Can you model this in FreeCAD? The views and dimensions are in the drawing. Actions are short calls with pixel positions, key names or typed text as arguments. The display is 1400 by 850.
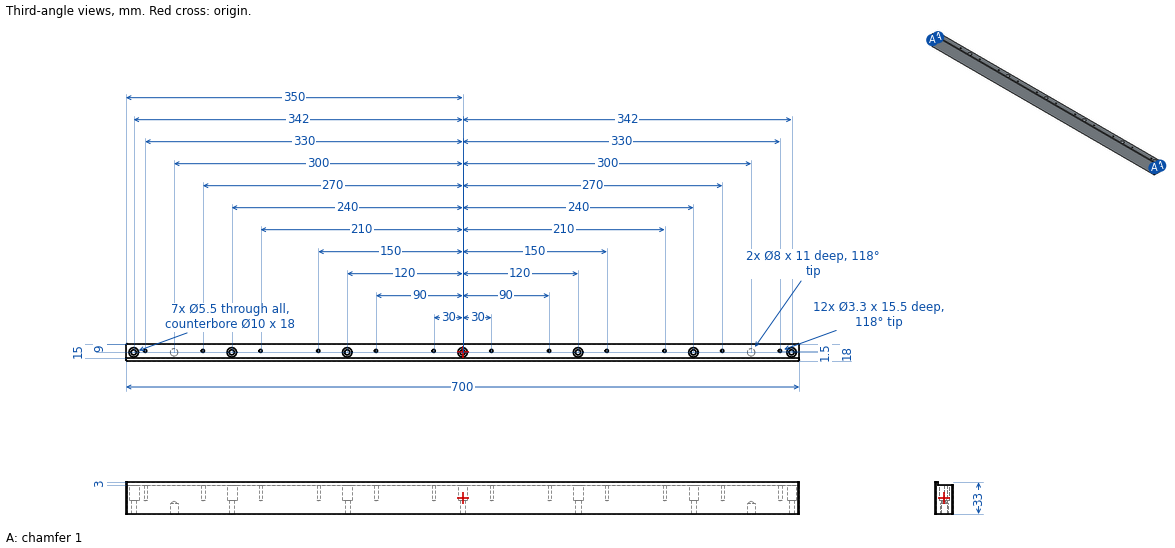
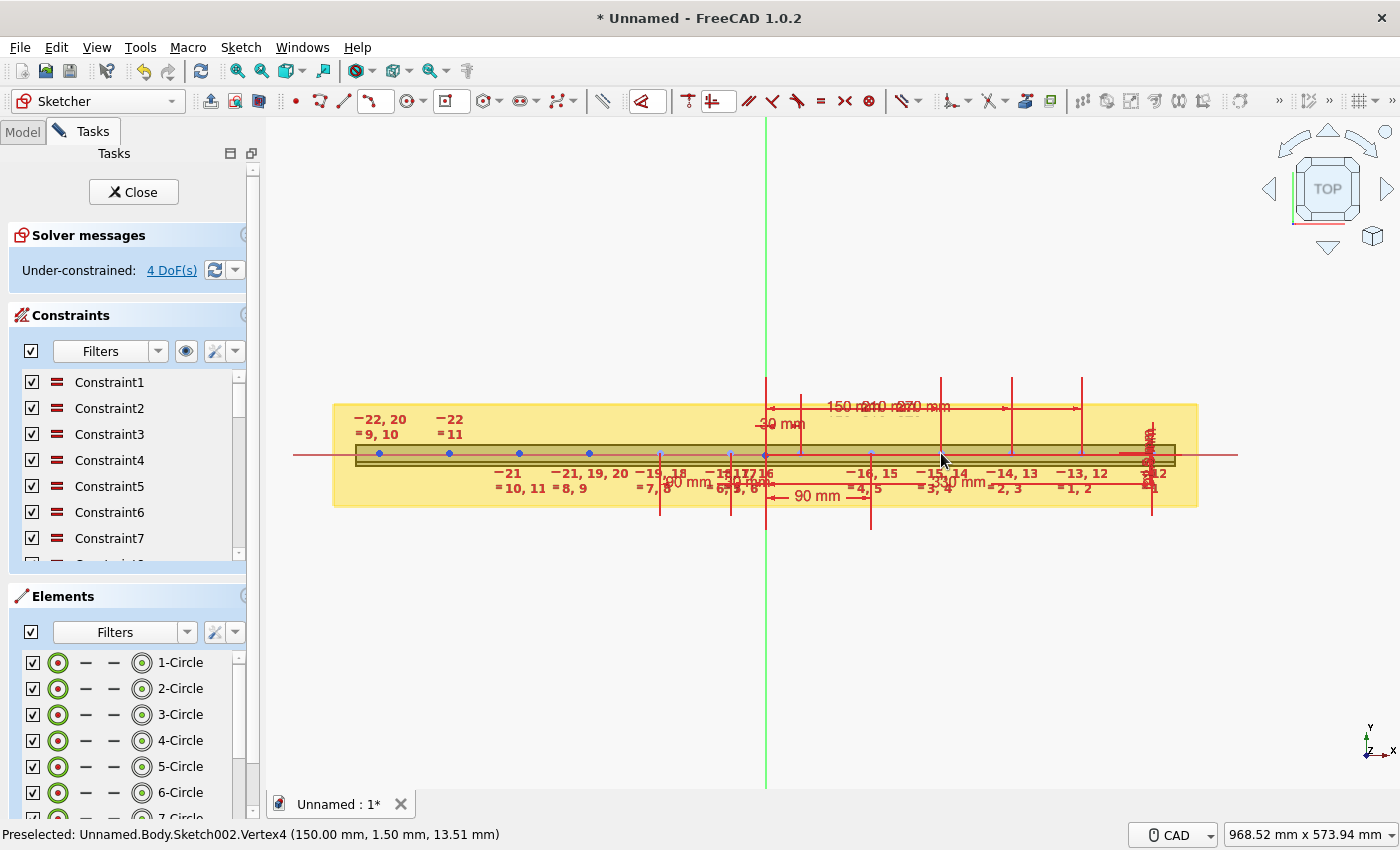
click(590, 453)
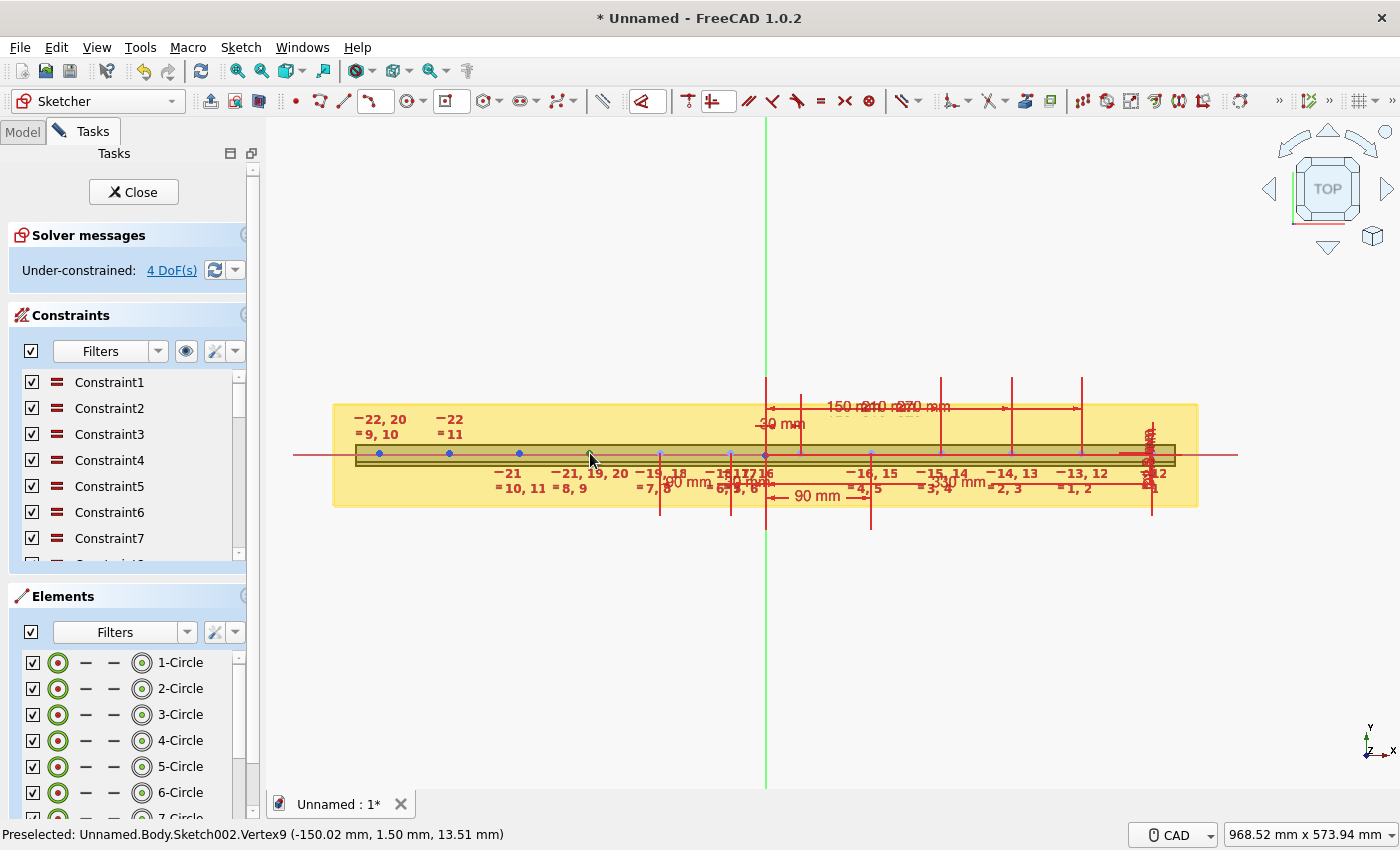
key(l)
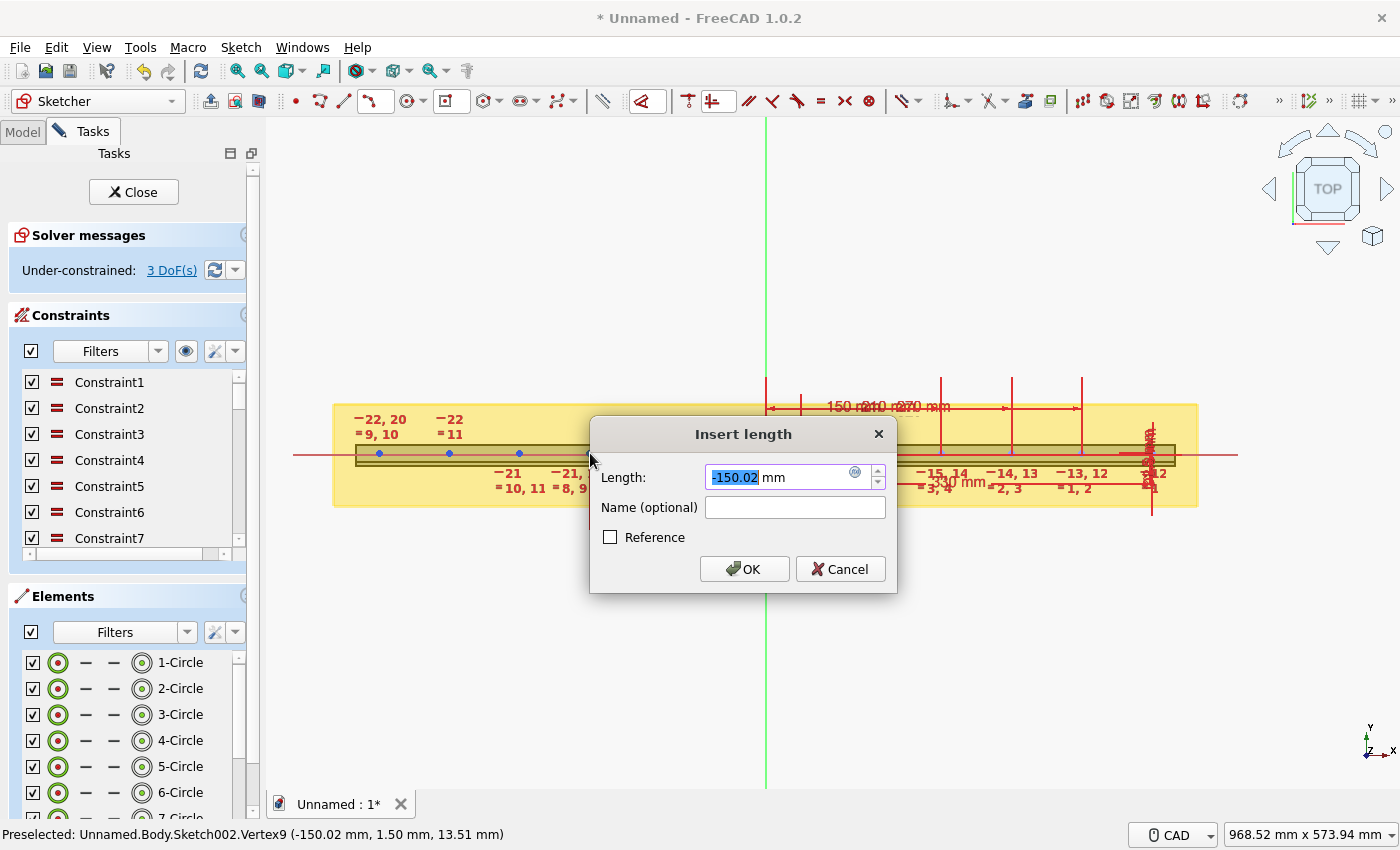
text(-150)
key(Return)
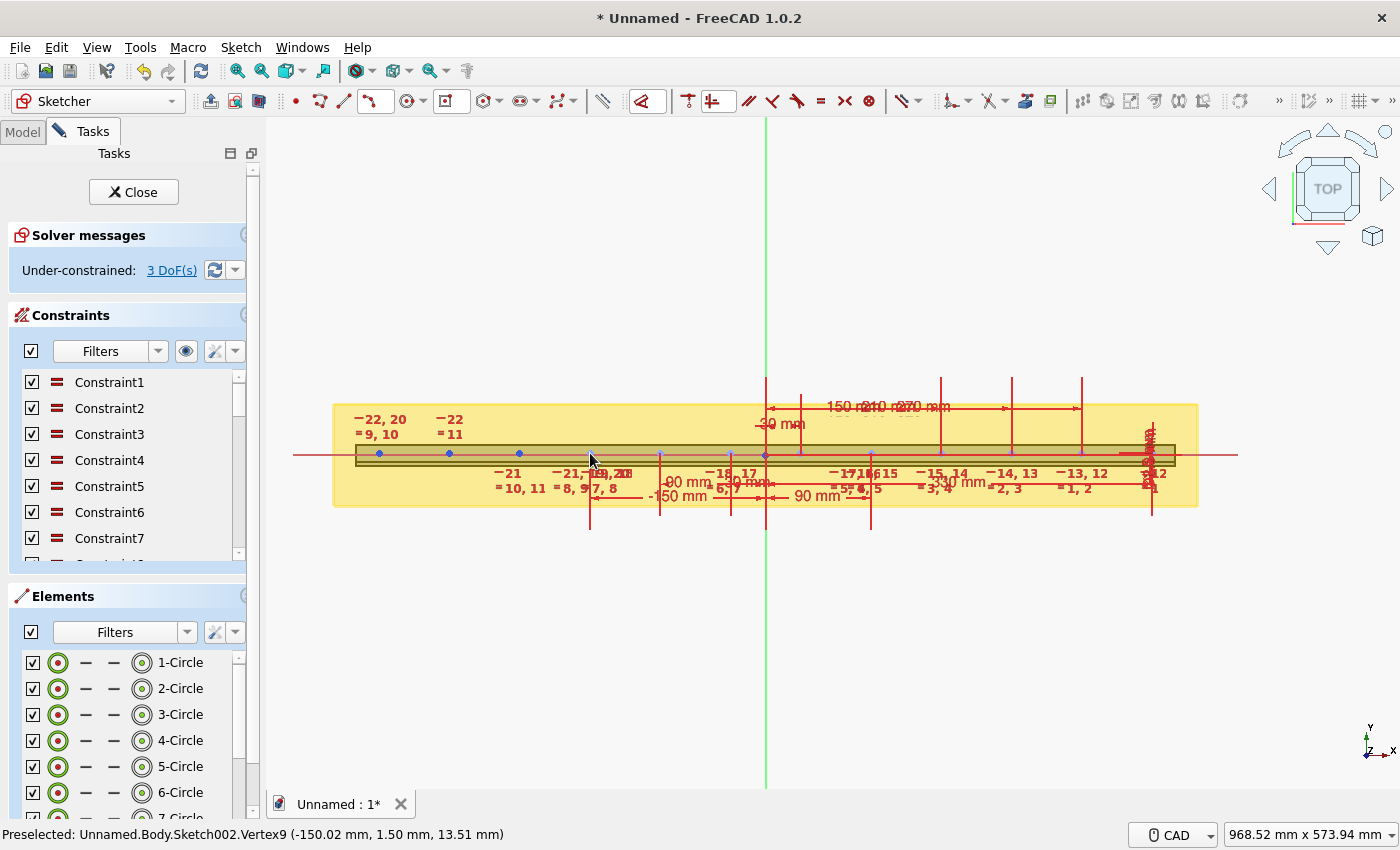
click(379, 453)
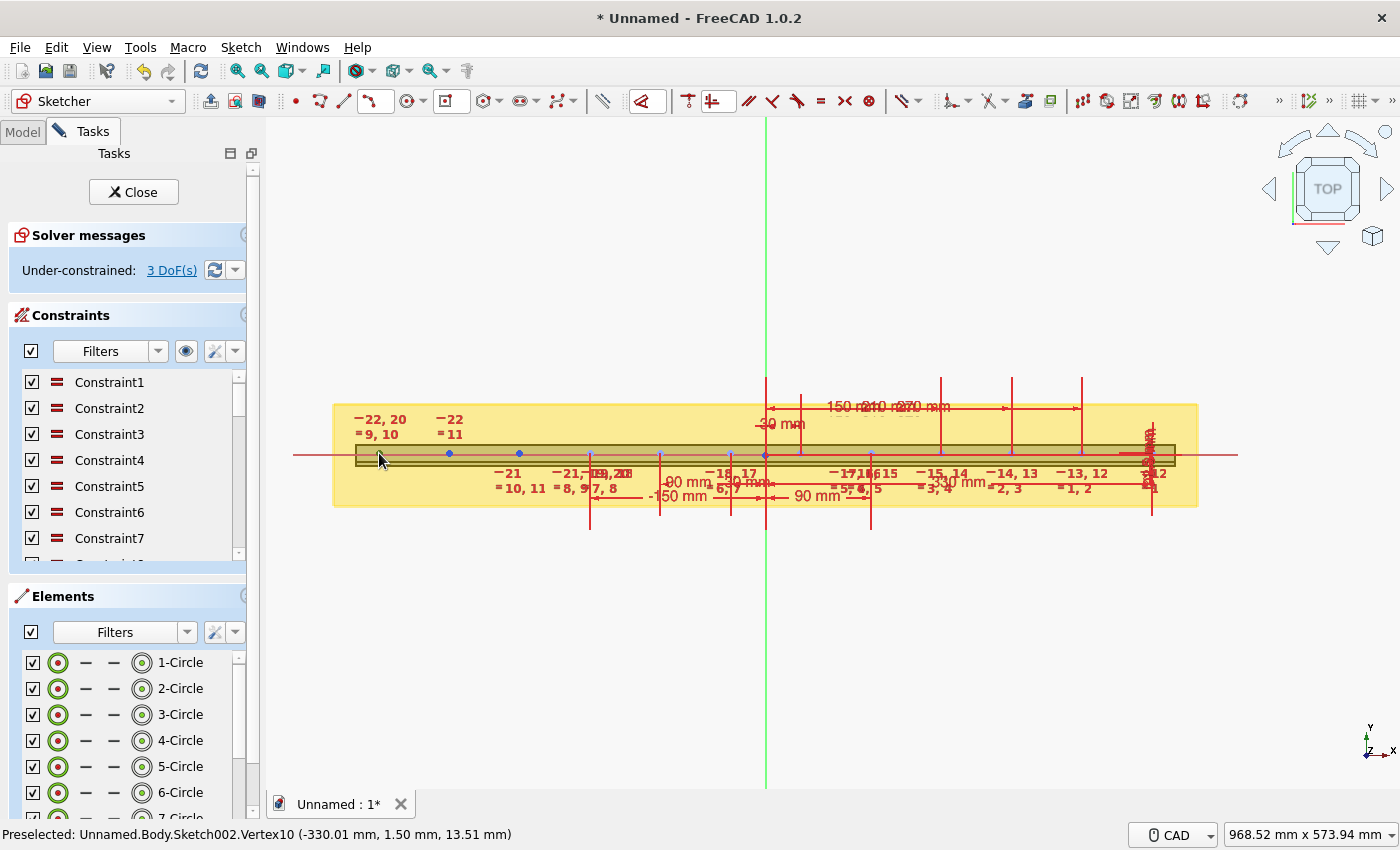
key(l)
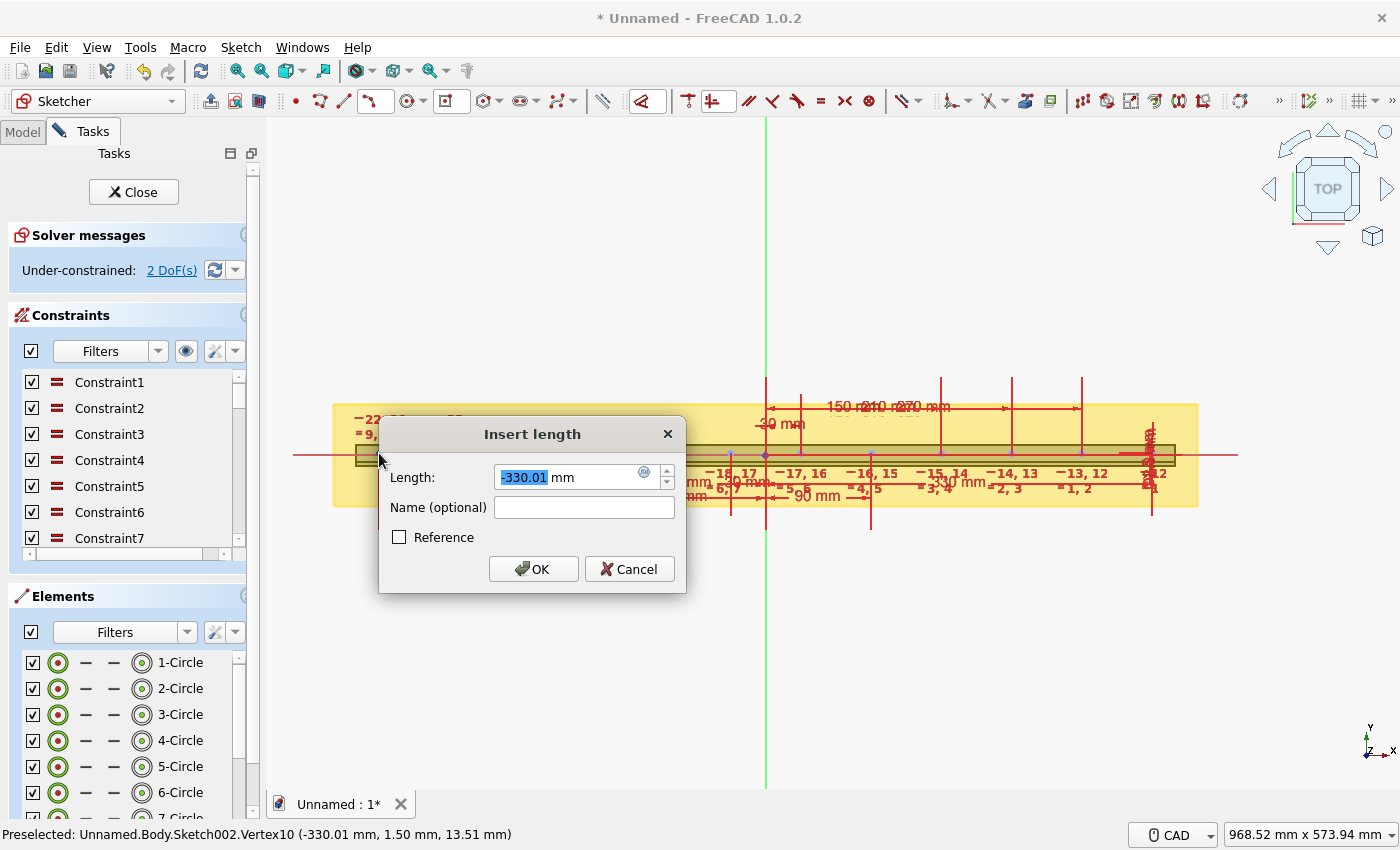
text(-330)
key(Return)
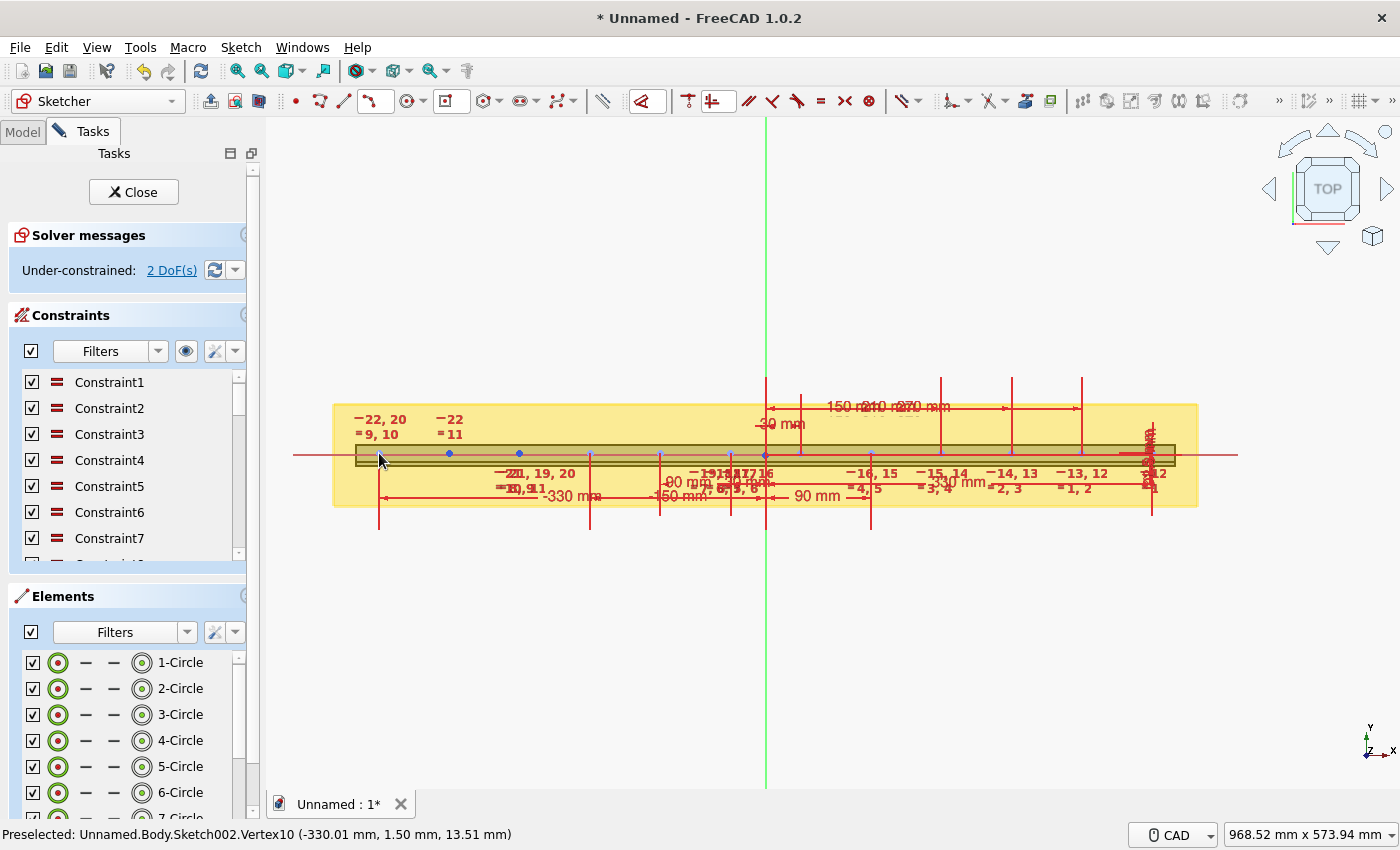
click(520, 453)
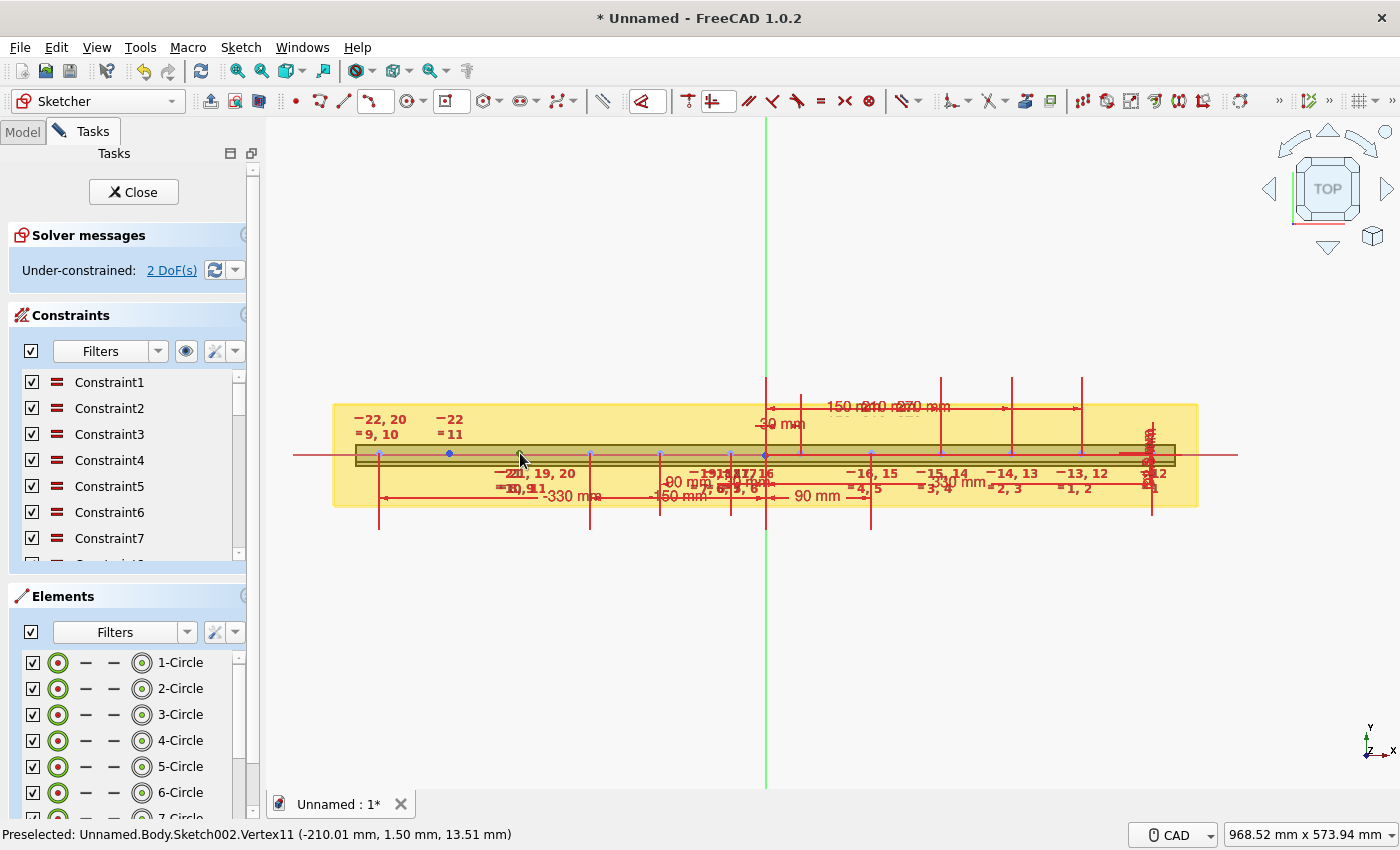
key(l)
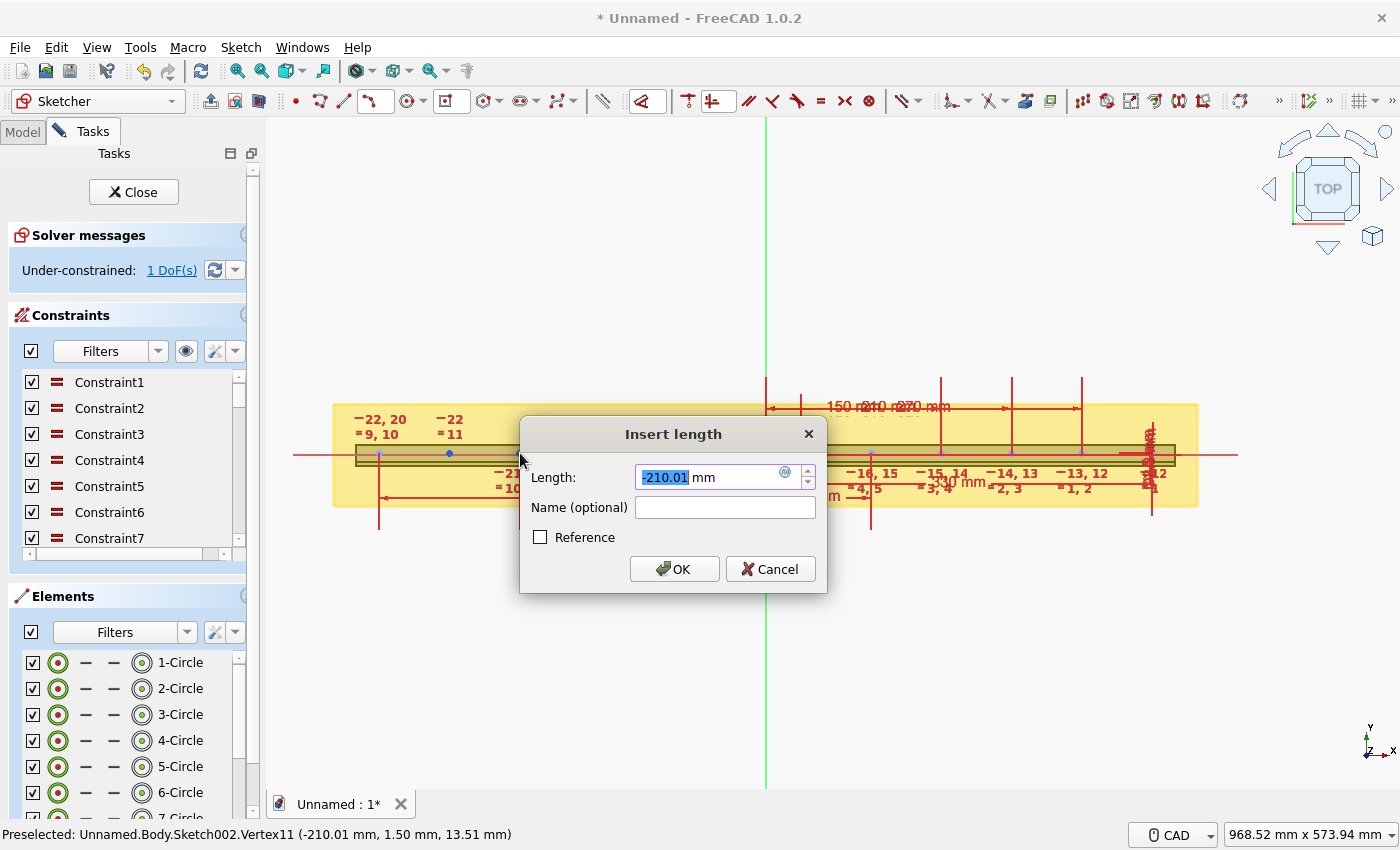
text(-210)
key(Return)